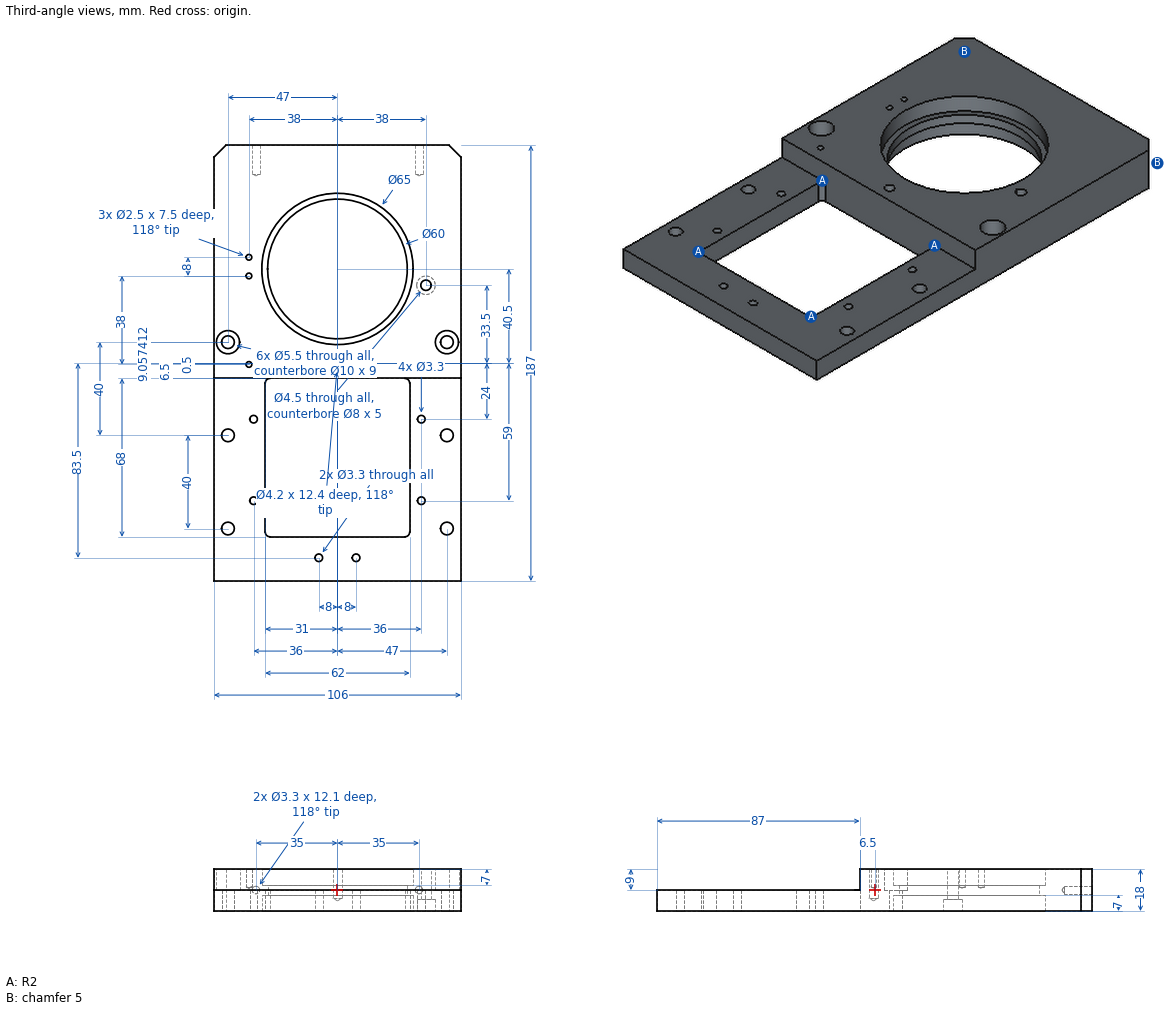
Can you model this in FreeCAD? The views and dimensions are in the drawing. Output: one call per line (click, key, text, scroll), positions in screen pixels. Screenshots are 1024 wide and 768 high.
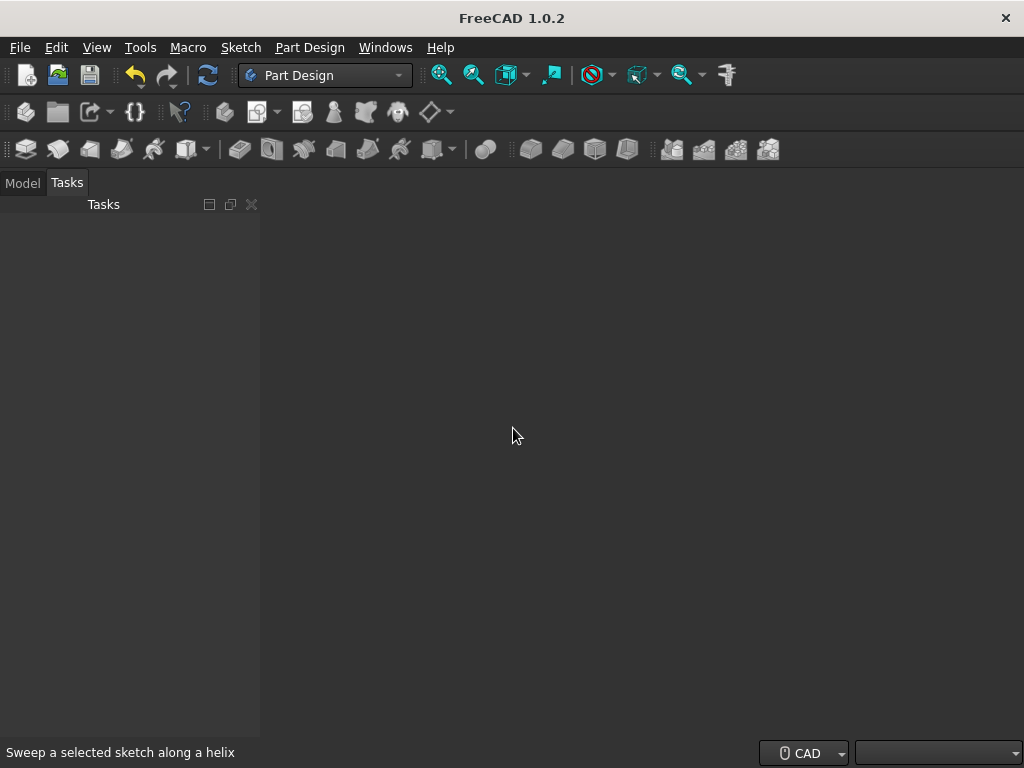
click(26, 76)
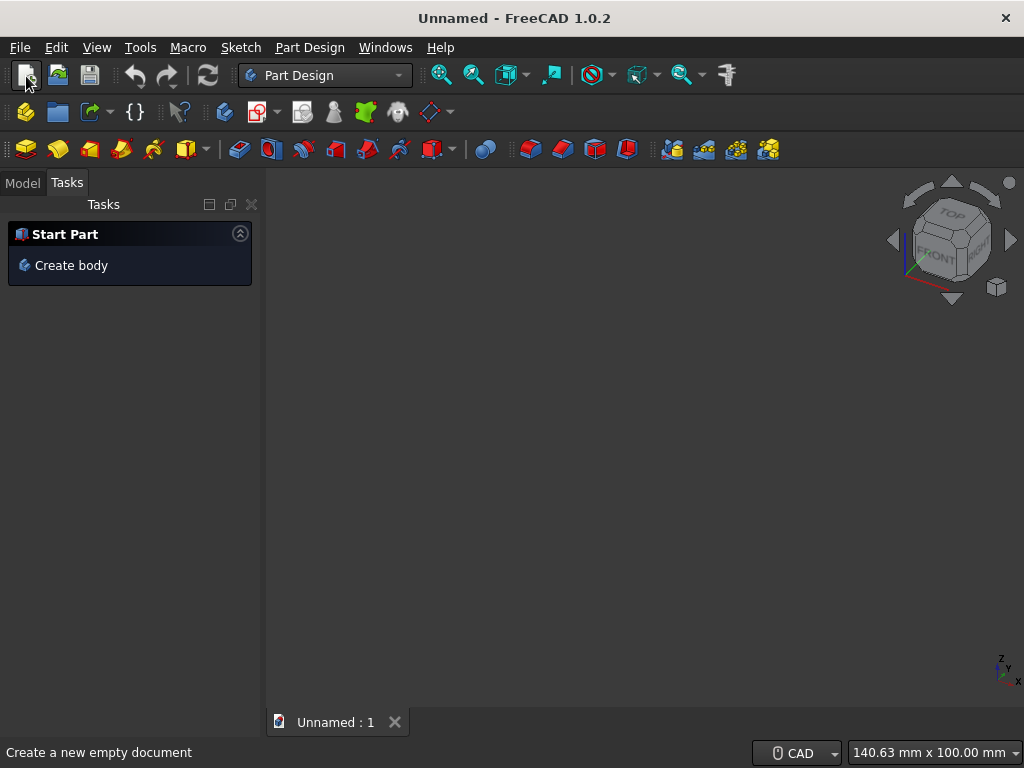
click(258, 112)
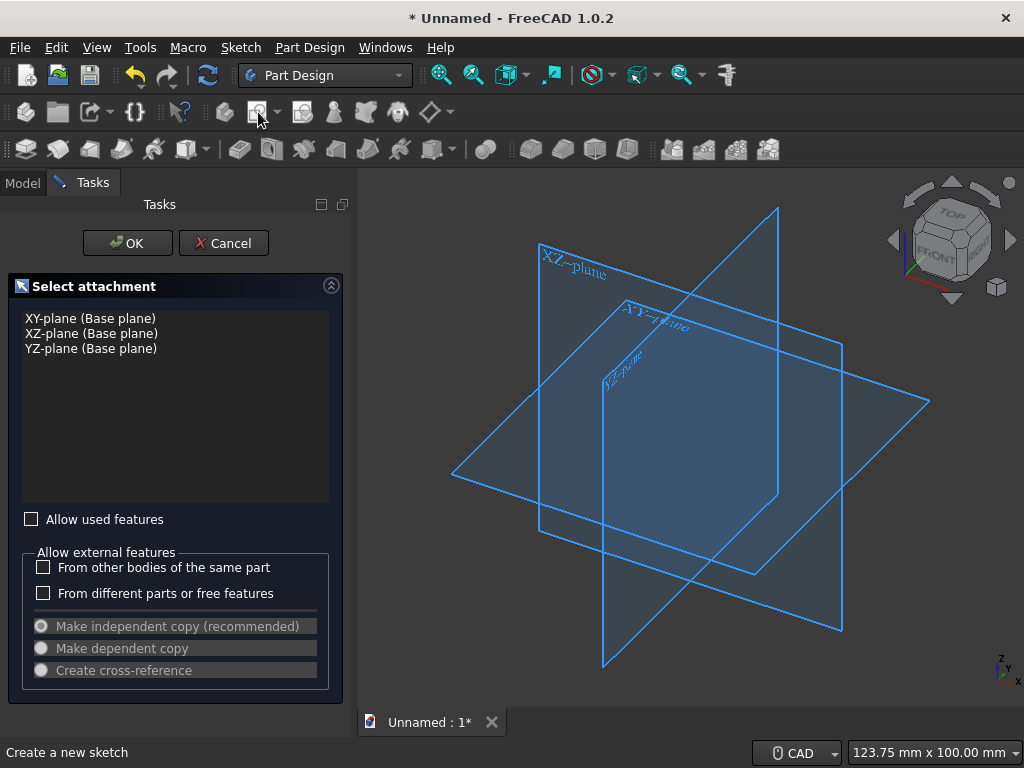
click(82, 318)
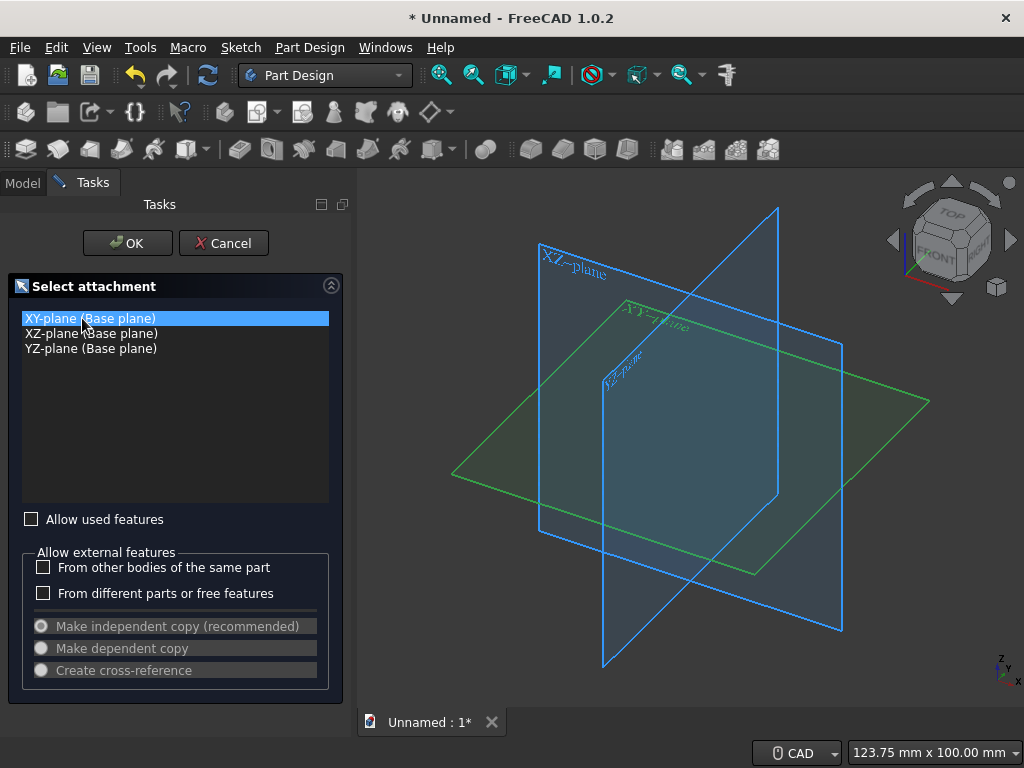
click(128, 243)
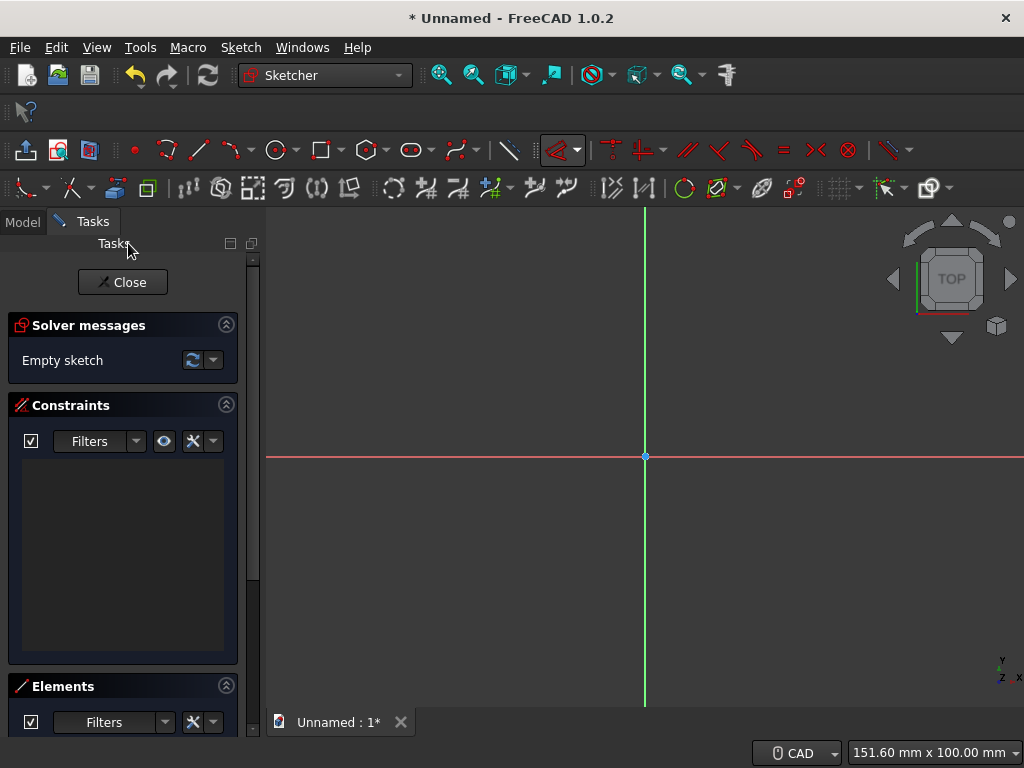
scroll(537, 457, down, 5)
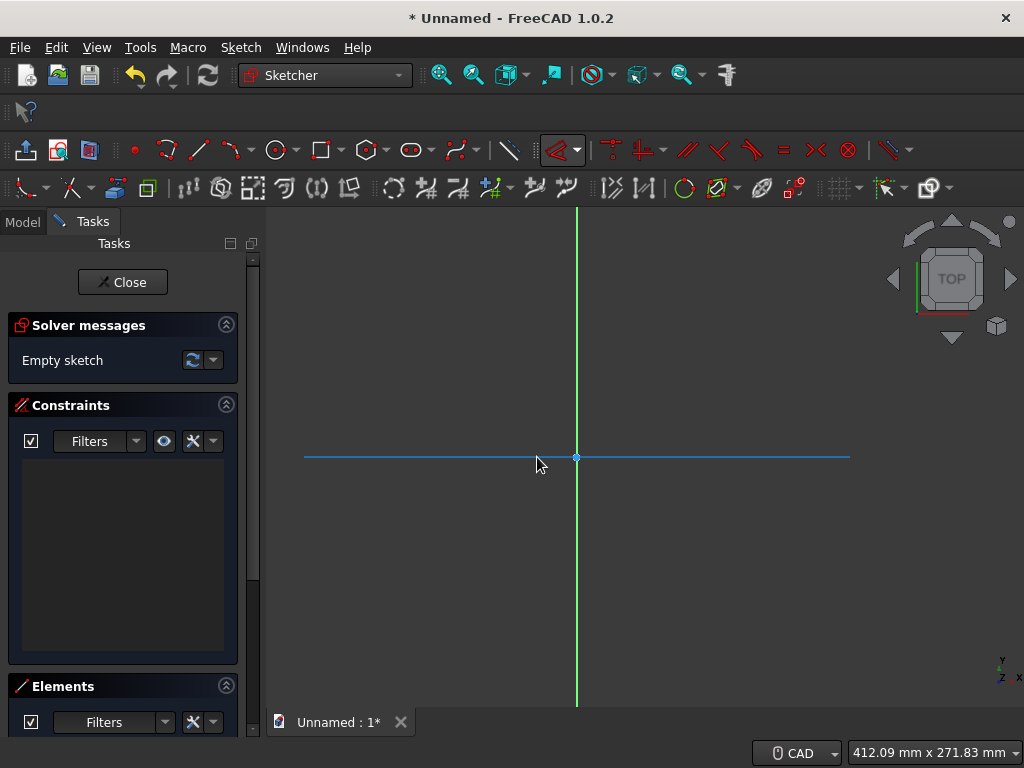
key(g)
key(v)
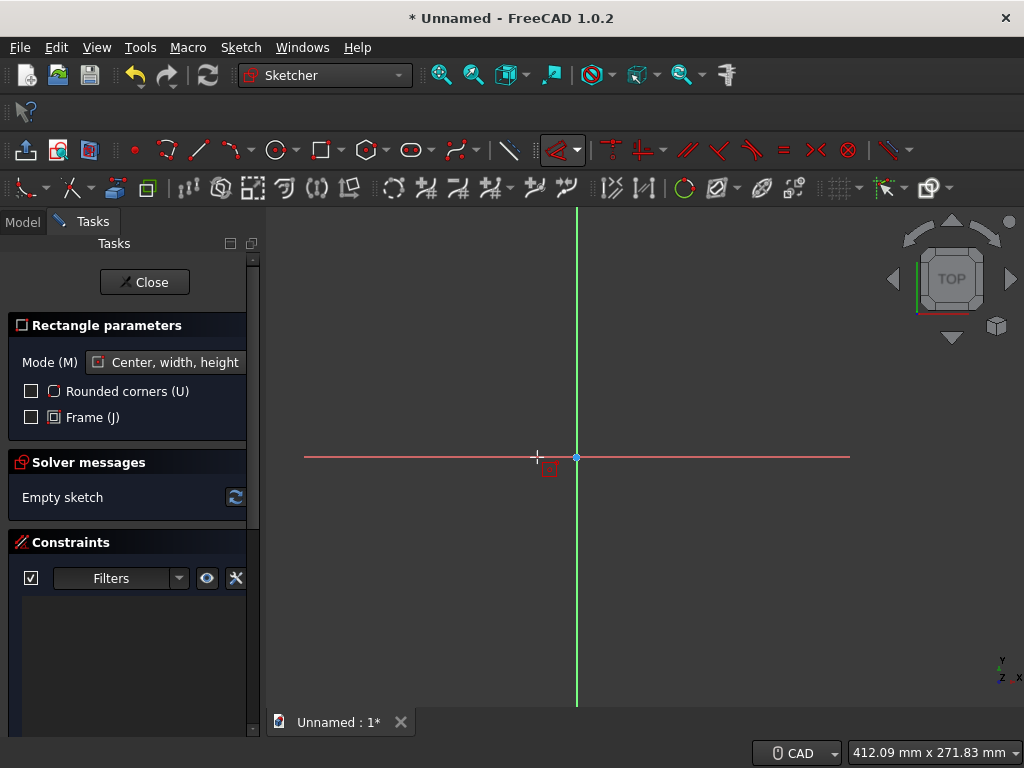
click(577, 457)
click(674, 285)
key(Escape)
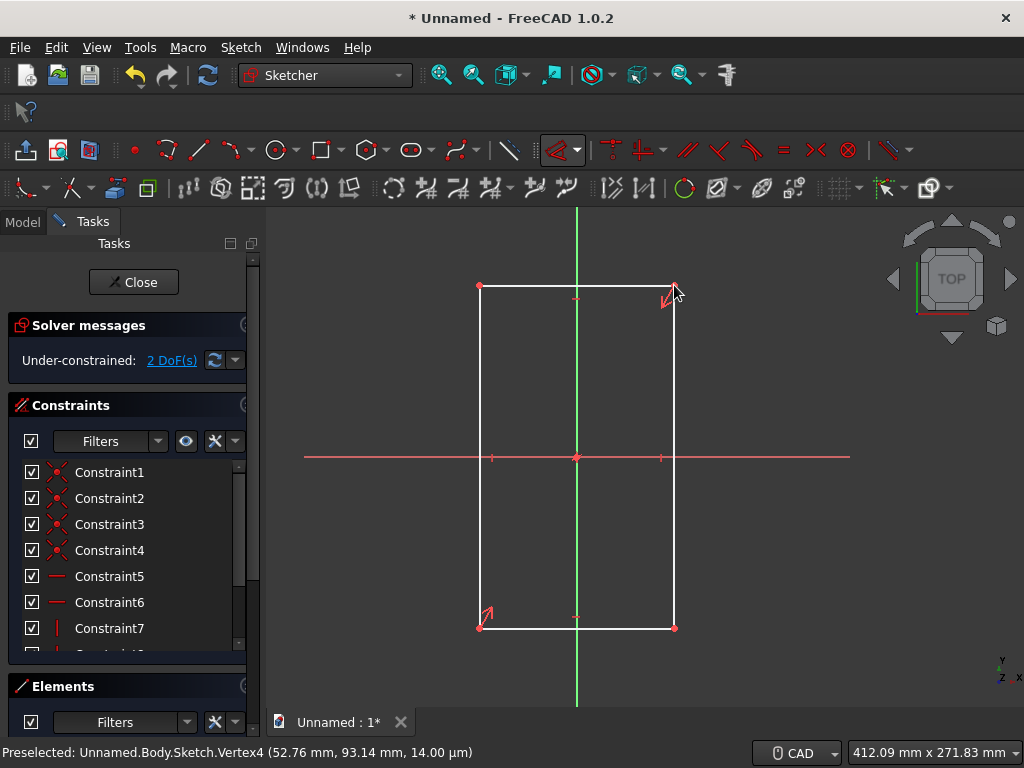
click(556, 150)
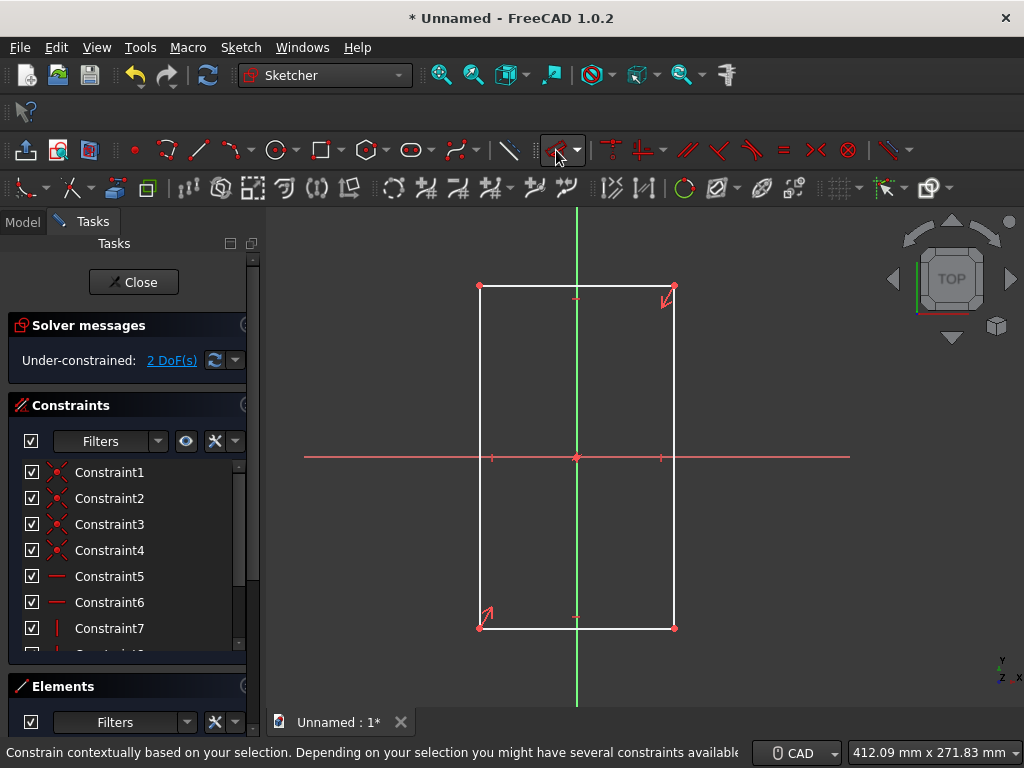
click(538, 629)
click(532, 663)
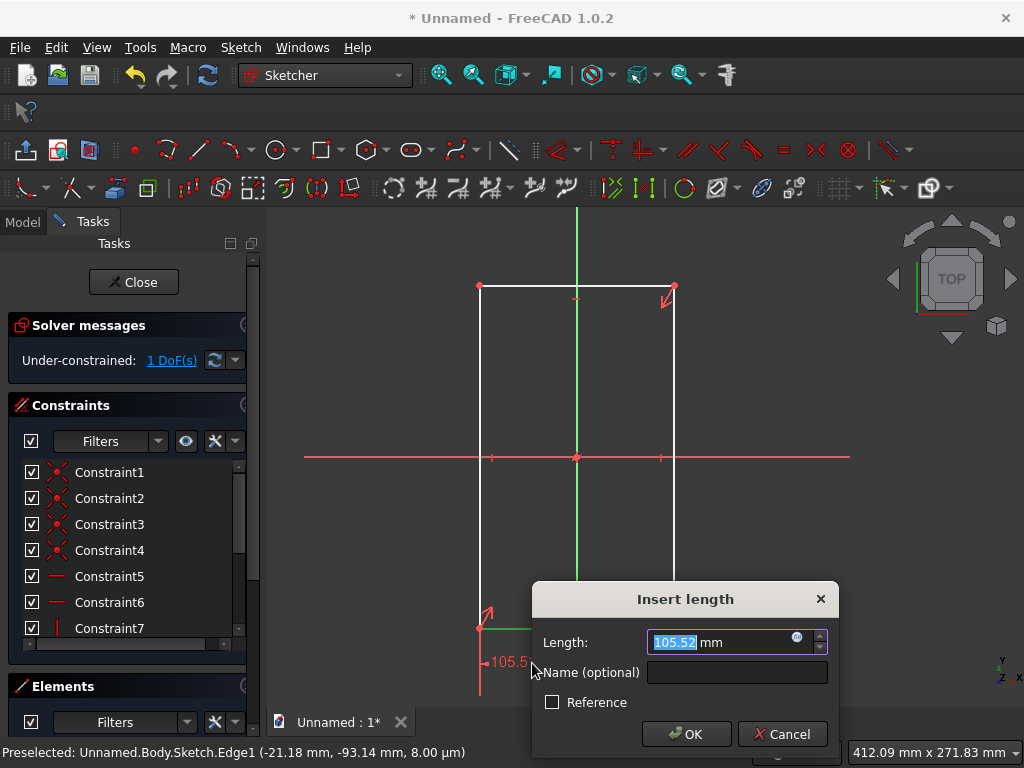
text(106)
key(Return)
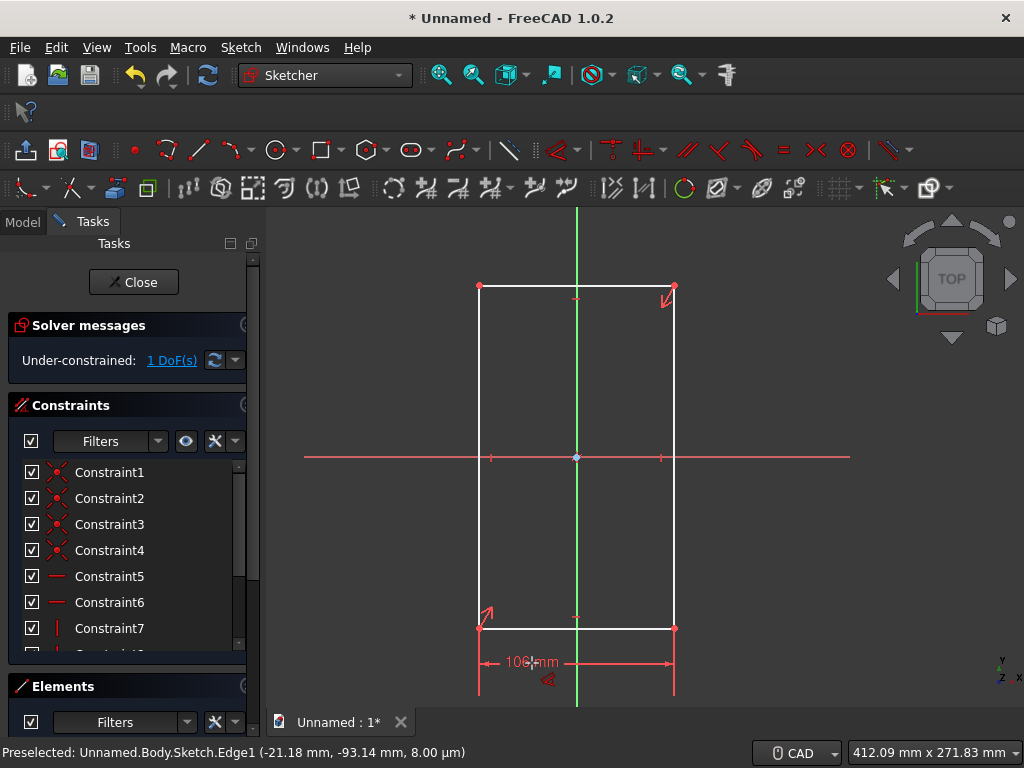
click(674, 526)
click(708, 379)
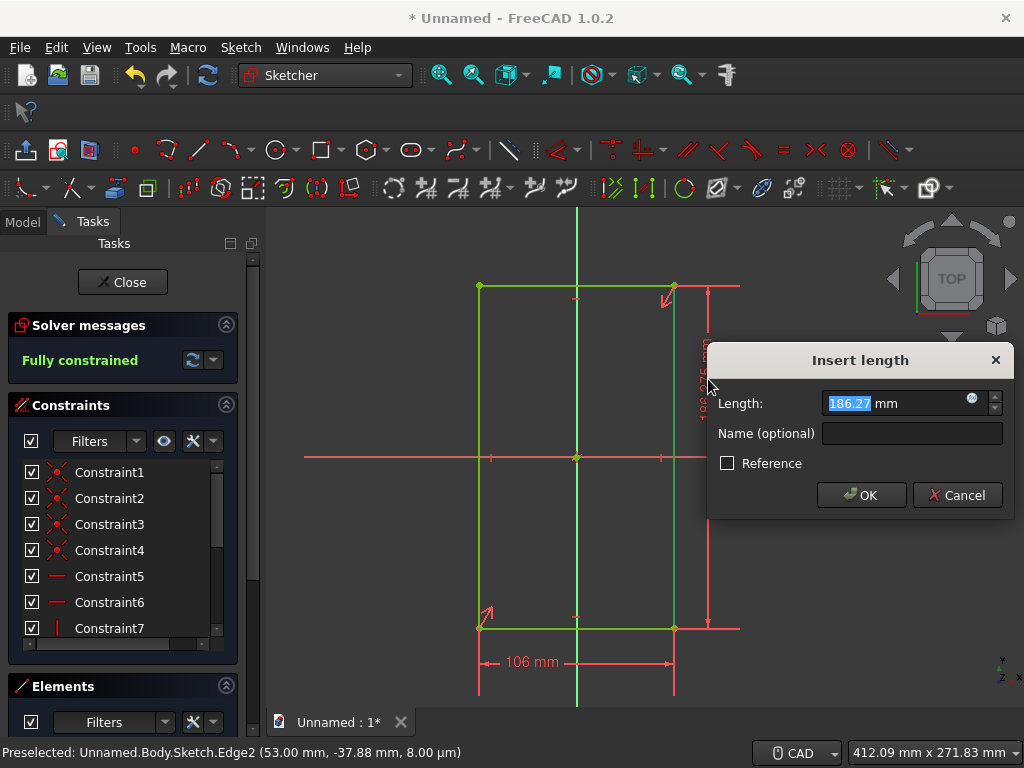
text(187)
key(Return)
key(Escape)